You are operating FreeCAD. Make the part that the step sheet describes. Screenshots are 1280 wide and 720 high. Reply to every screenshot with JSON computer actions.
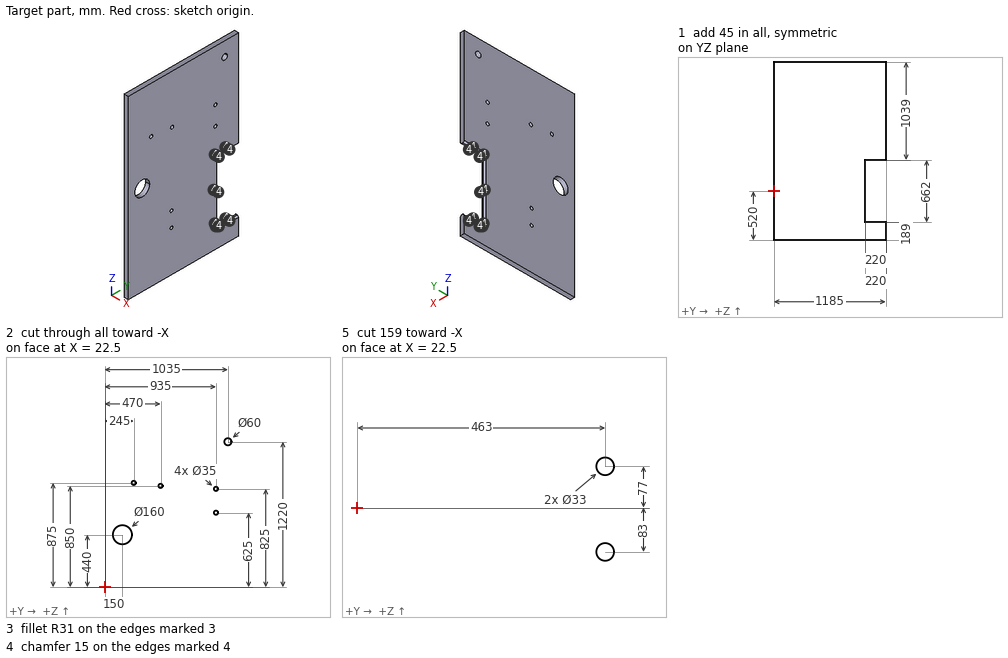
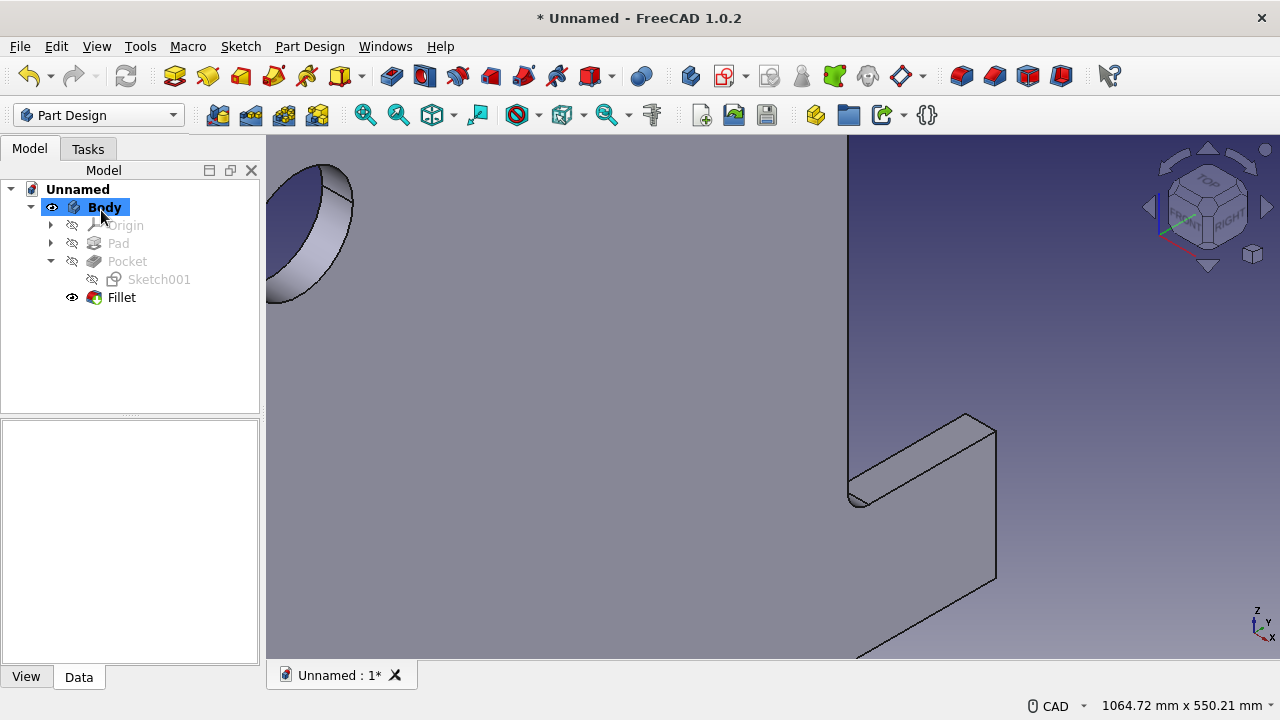
{"action": "left_click", "coordinate": [366, 116]}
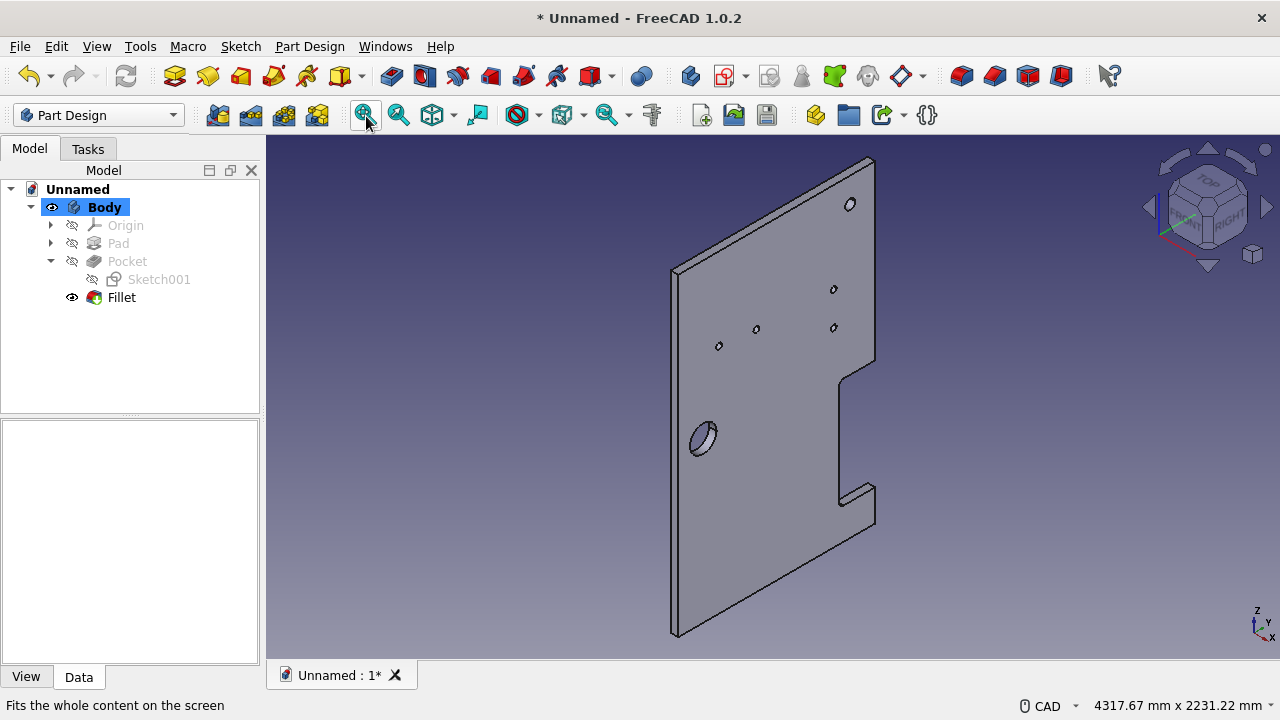
{"action": "left_click", "coordinate": [859, 495]}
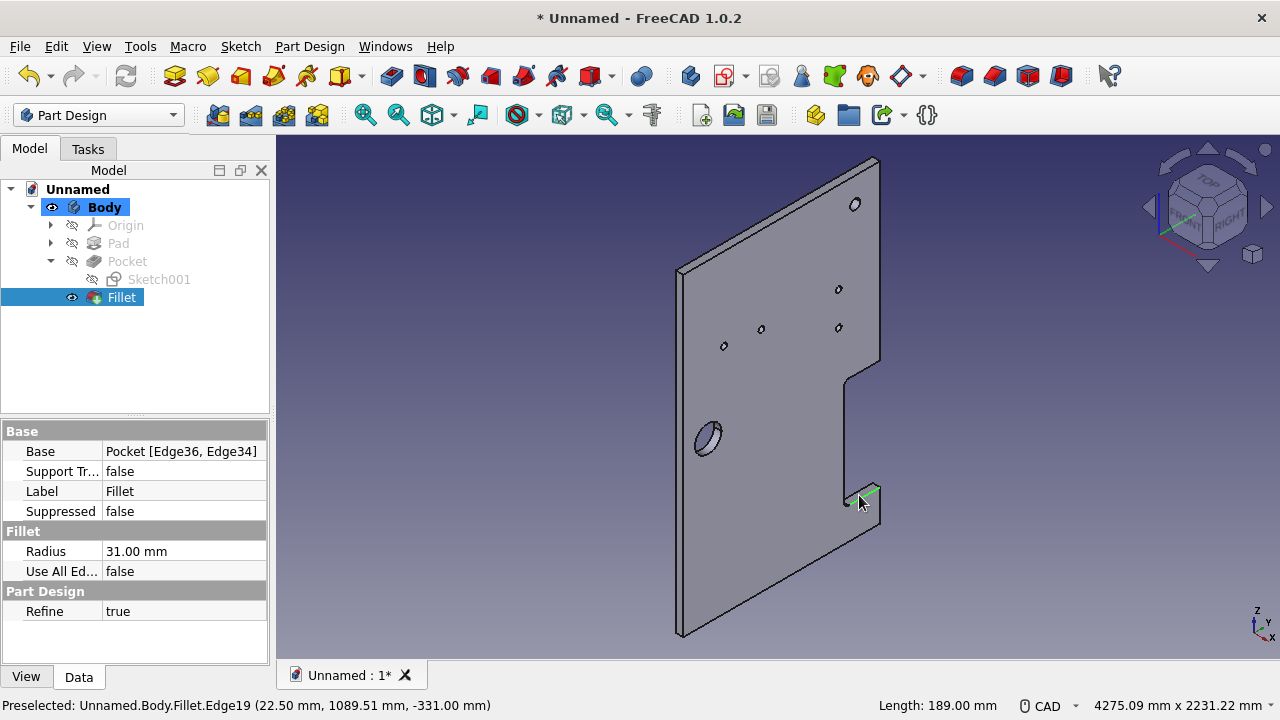
{"action": "left_click", "coordinate": [849, 505], "text": "ctrl"}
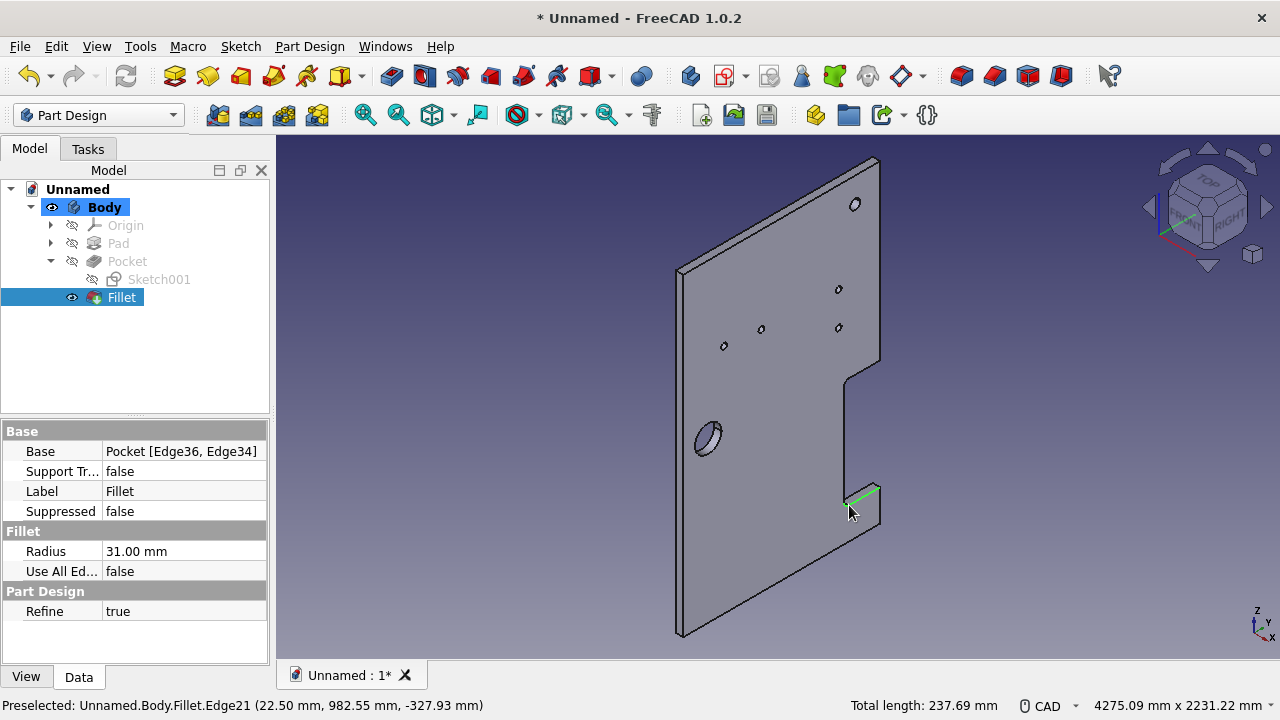
{"action": "key", "text": "2"}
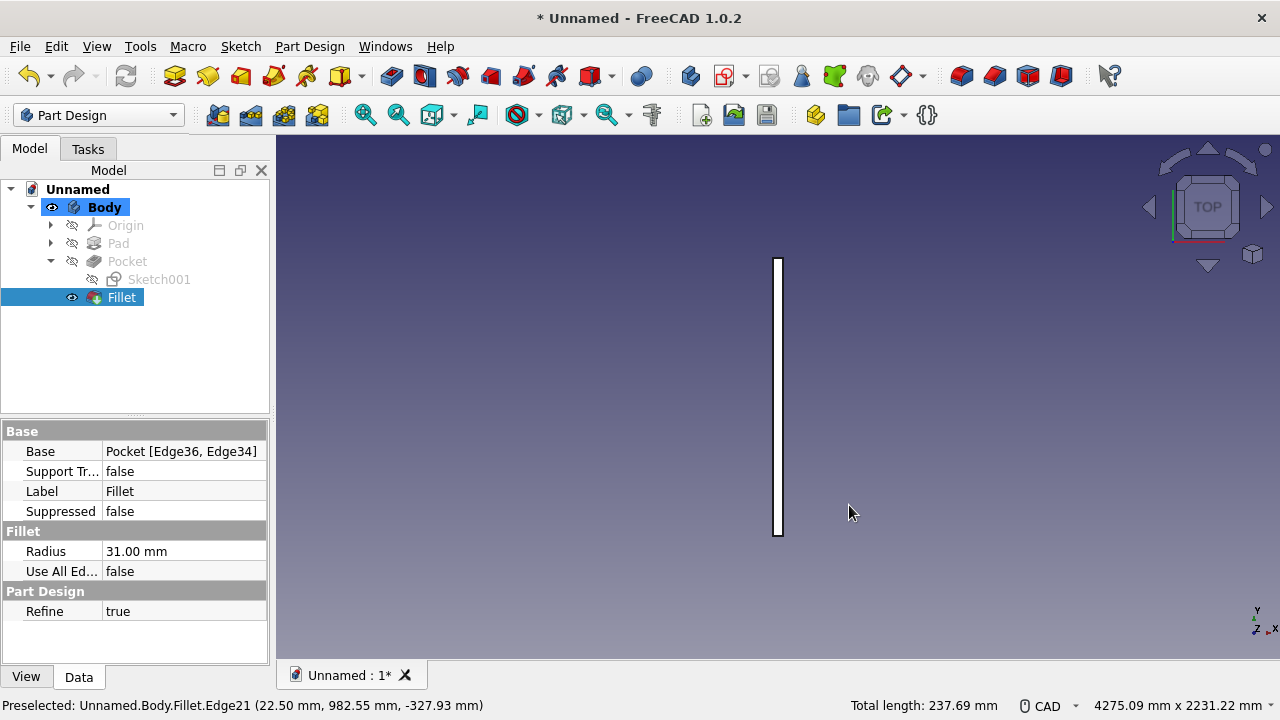
{"action": "key", "text": "0"}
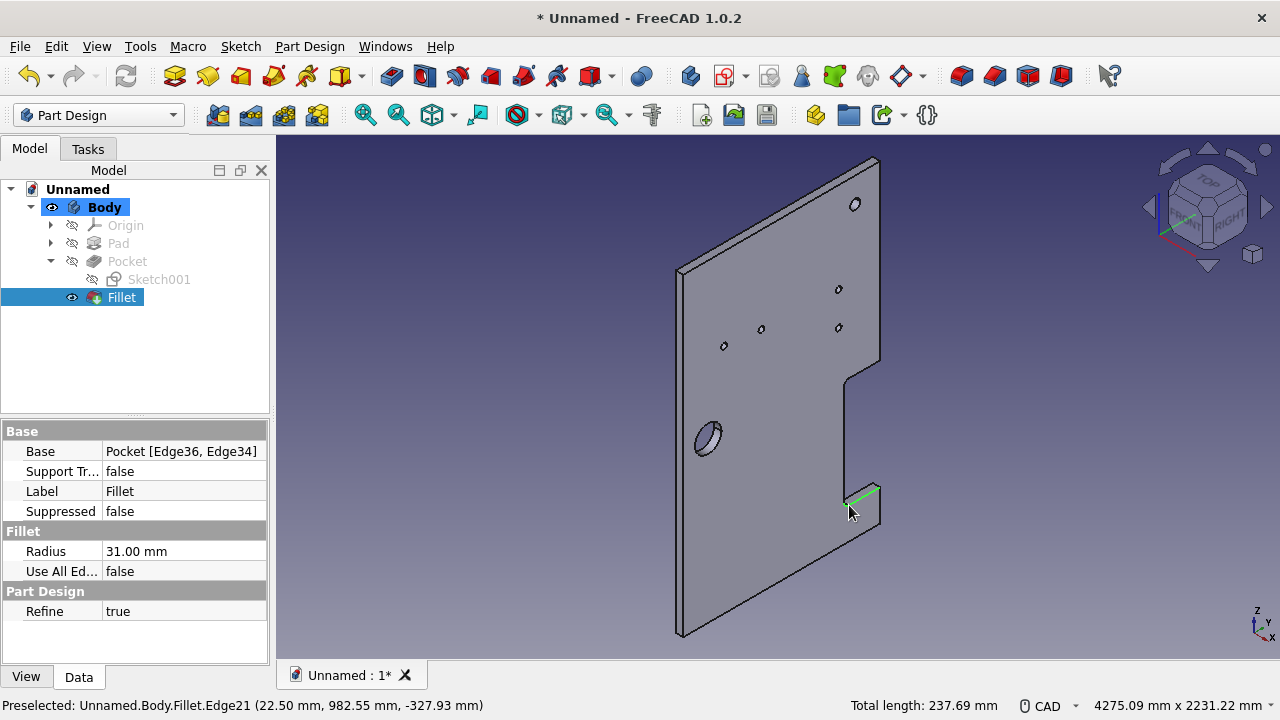
{"action": "key", "text": "1"}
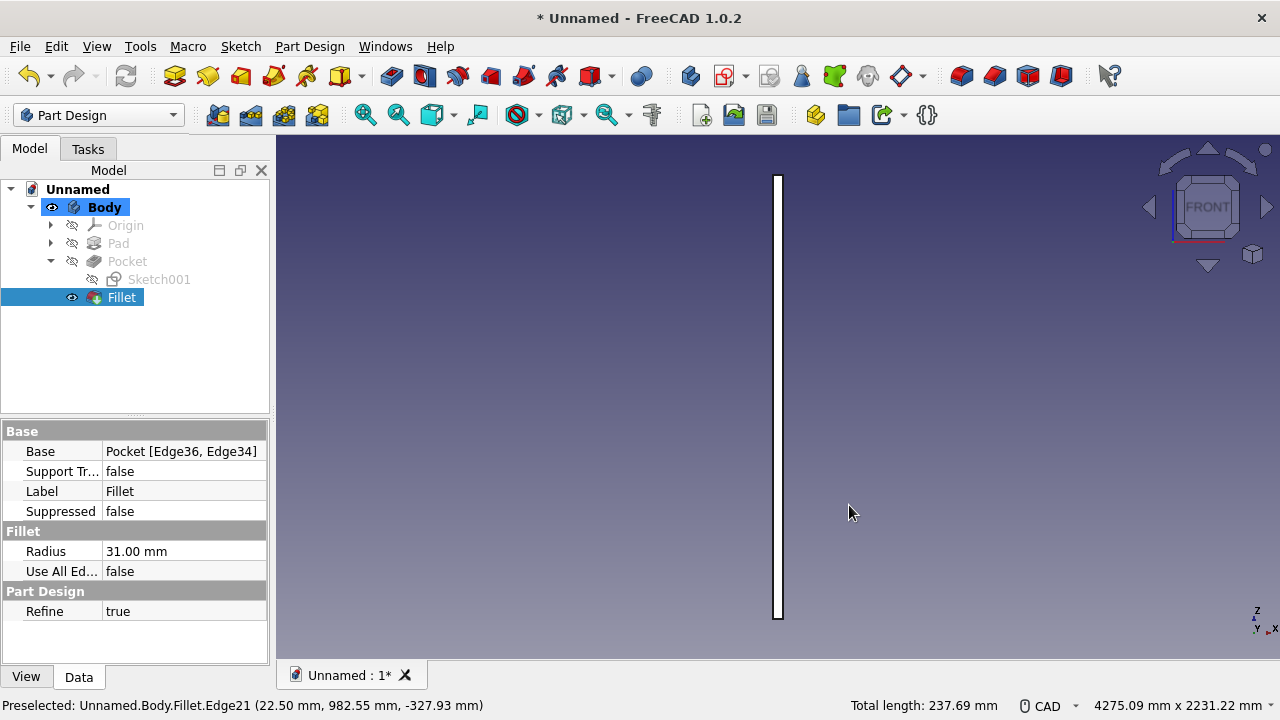
{"action": "key", "text": "3"}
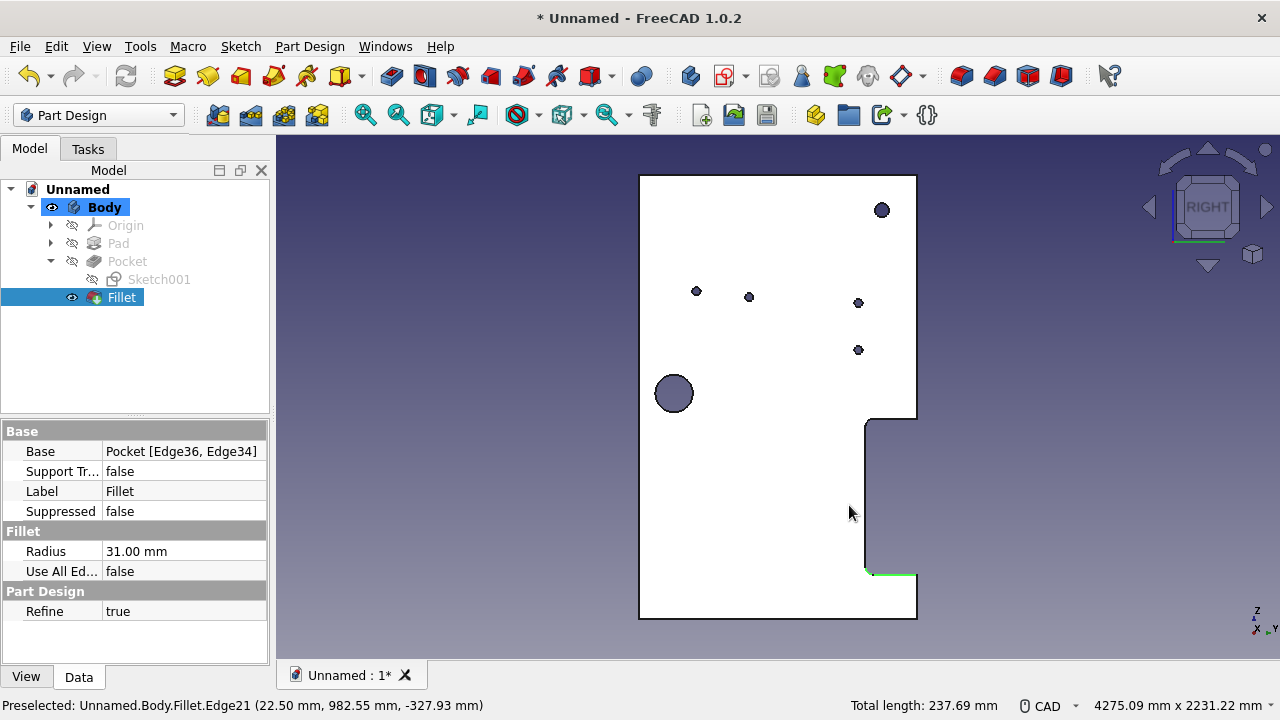
{"action": "left_click", "coordinate": [865, 496], "text": "ctrl"}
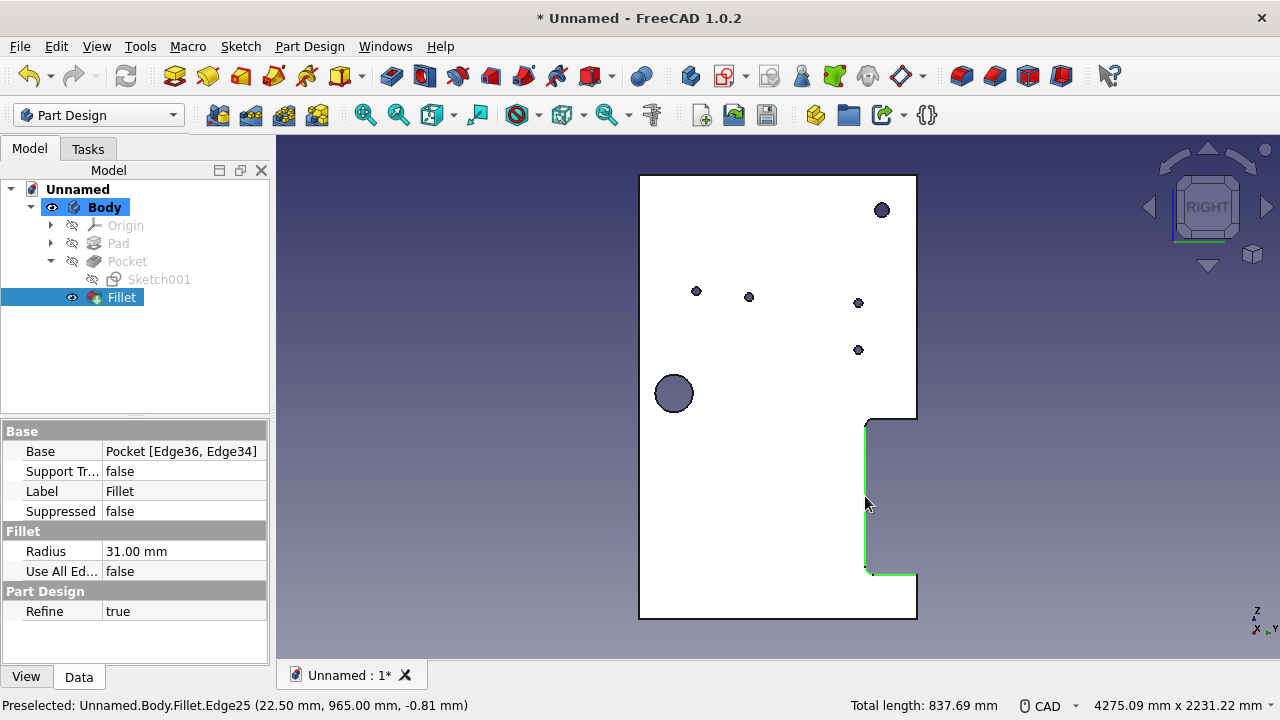
{"action": "left_click", "coordinate": [895, 418], "text": "ctrl"}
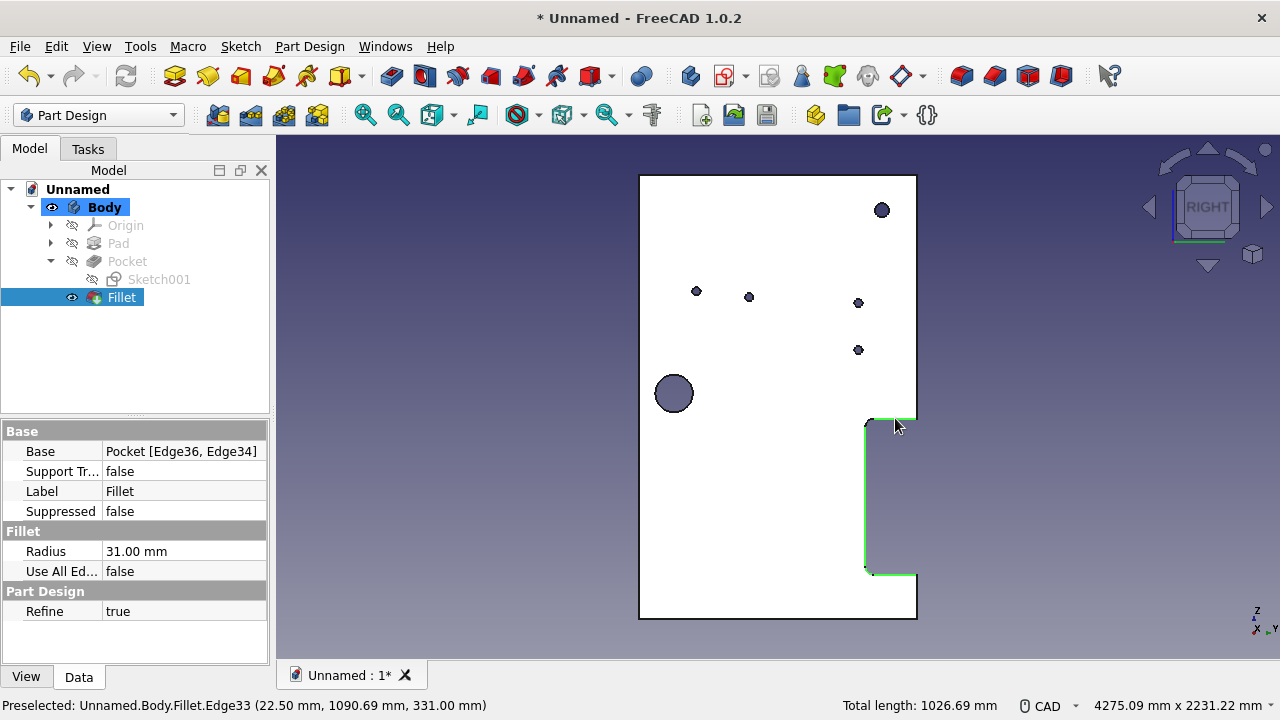
{"action": "key", "text": "5"}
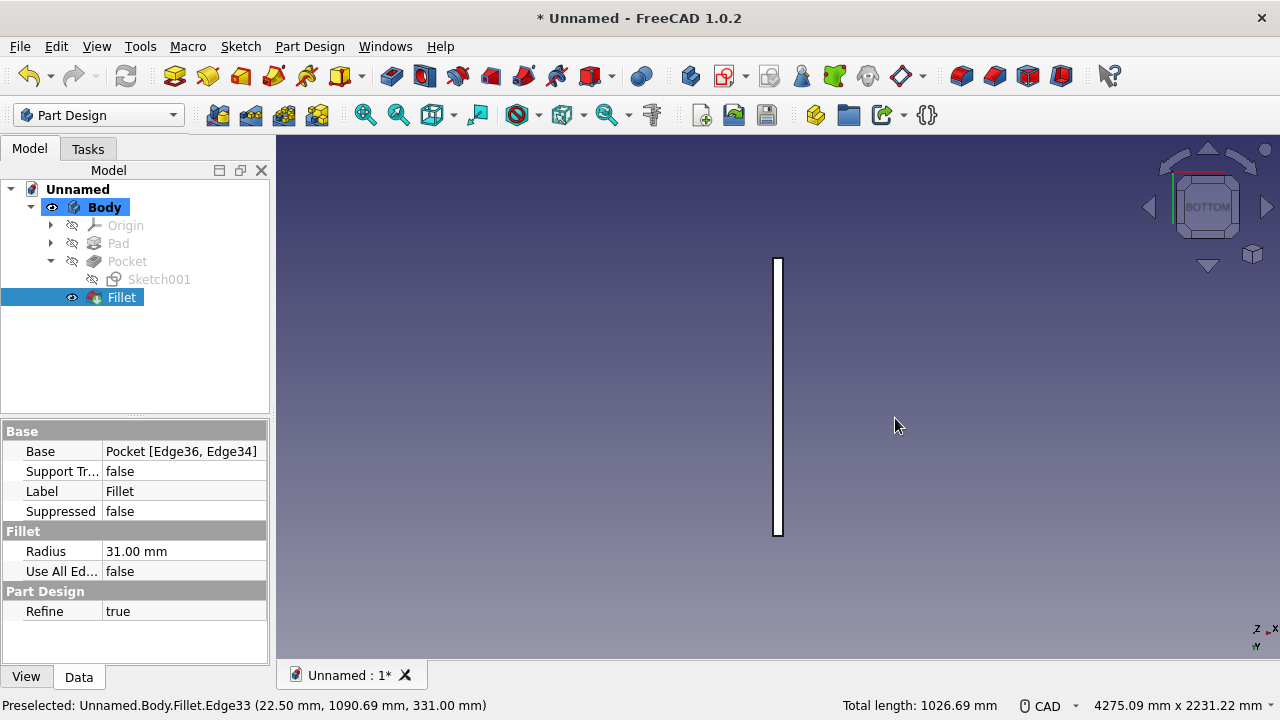
{"action": "key", "text": "4"}